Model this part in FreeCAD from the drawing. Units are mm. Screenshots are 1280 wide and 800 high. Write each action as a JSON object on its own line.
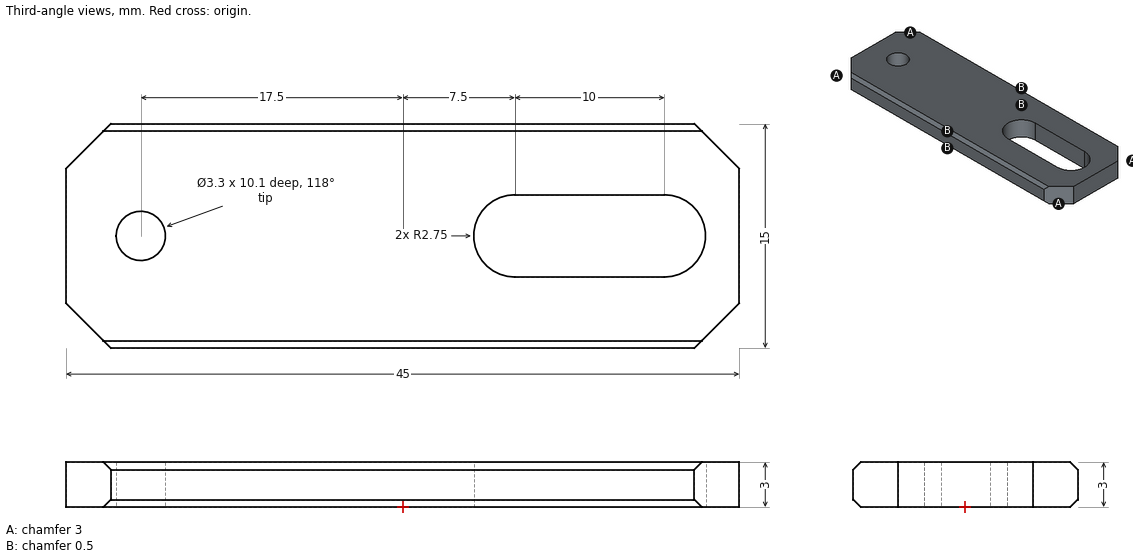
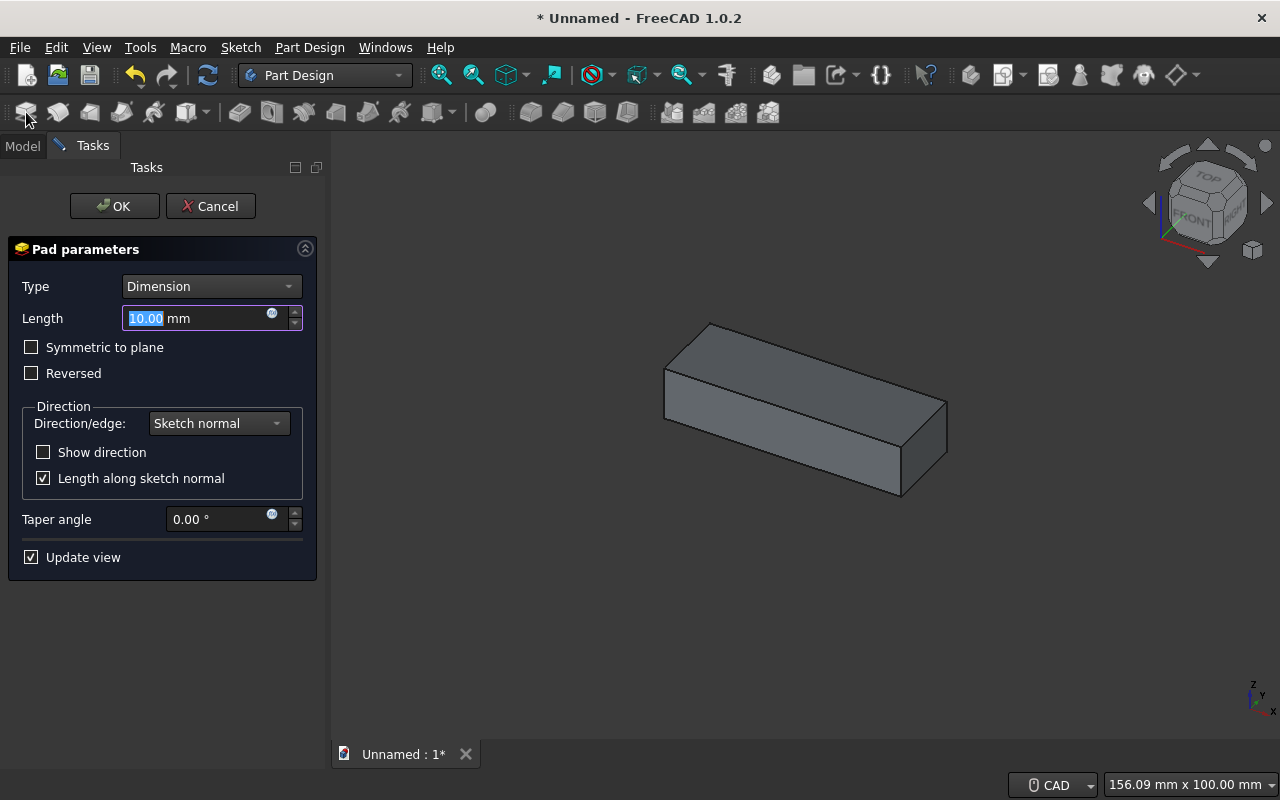
{"action": "type", "text": "3"}
{"action": "key", "text": "Tab"}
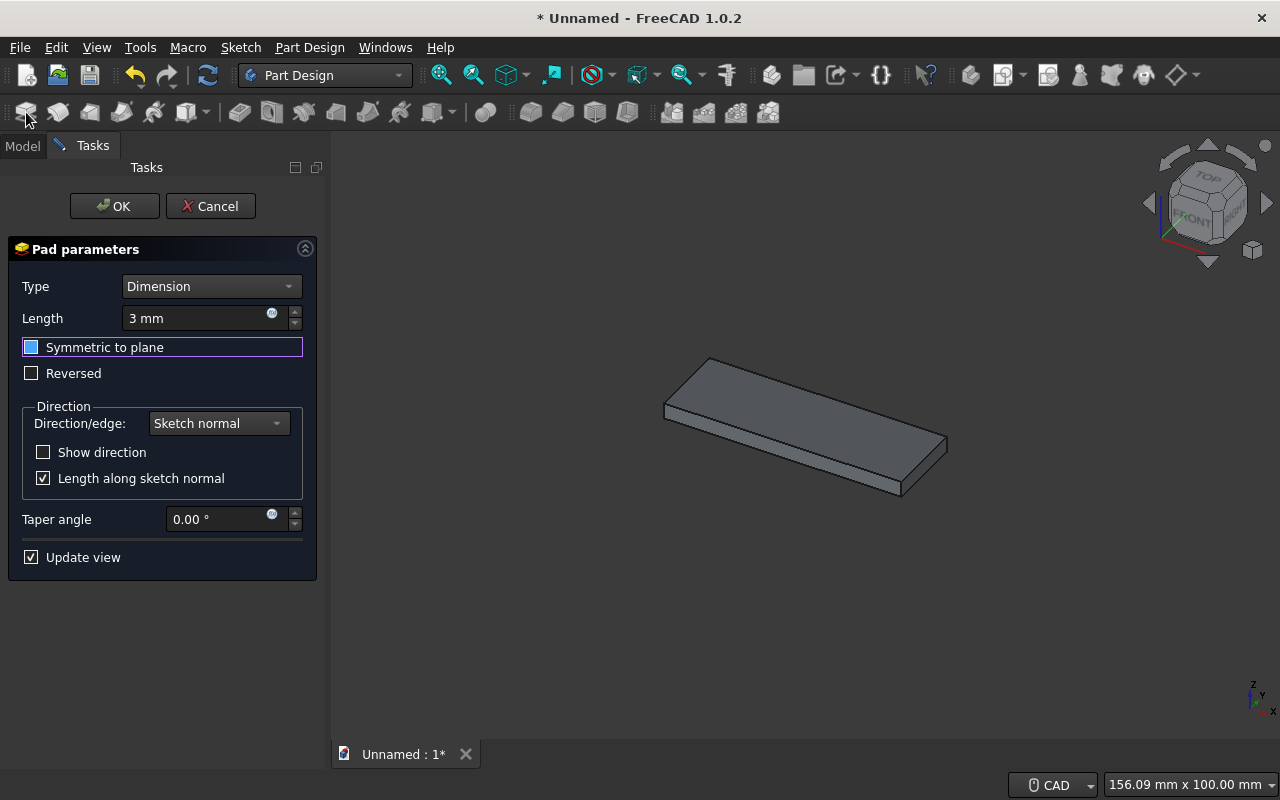
{"action": "left_click", "coordinate": [115, 206]}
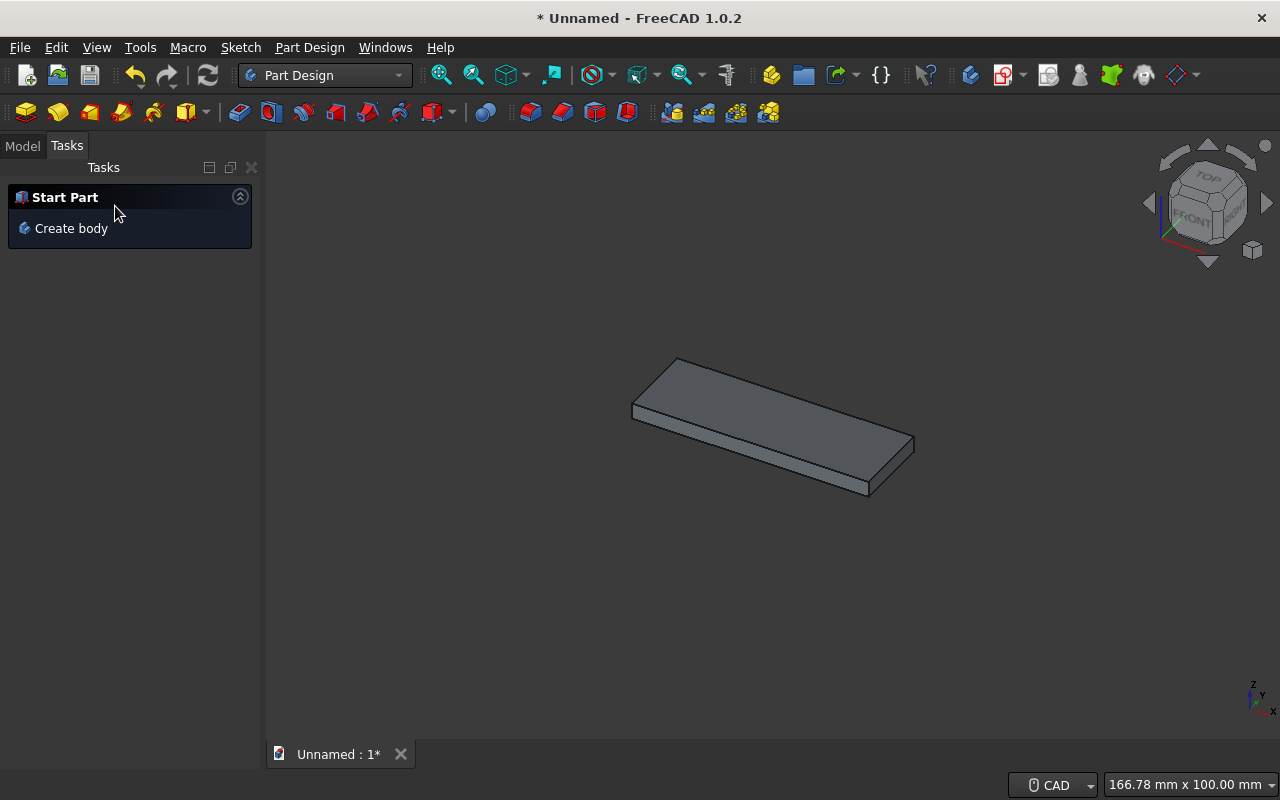
{"action": "left_click", "coordinate": [442, 76]}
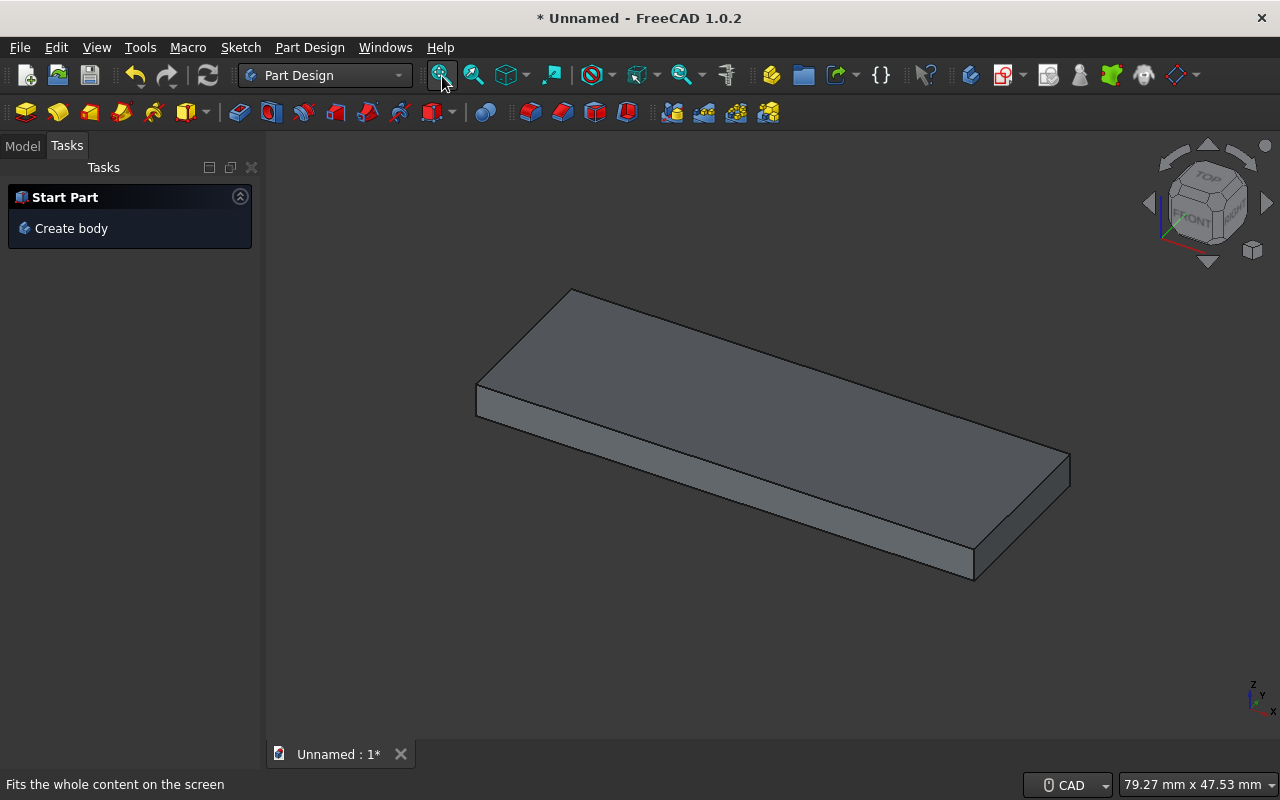
{"action": "left_click", "coordinate": [915, 465]}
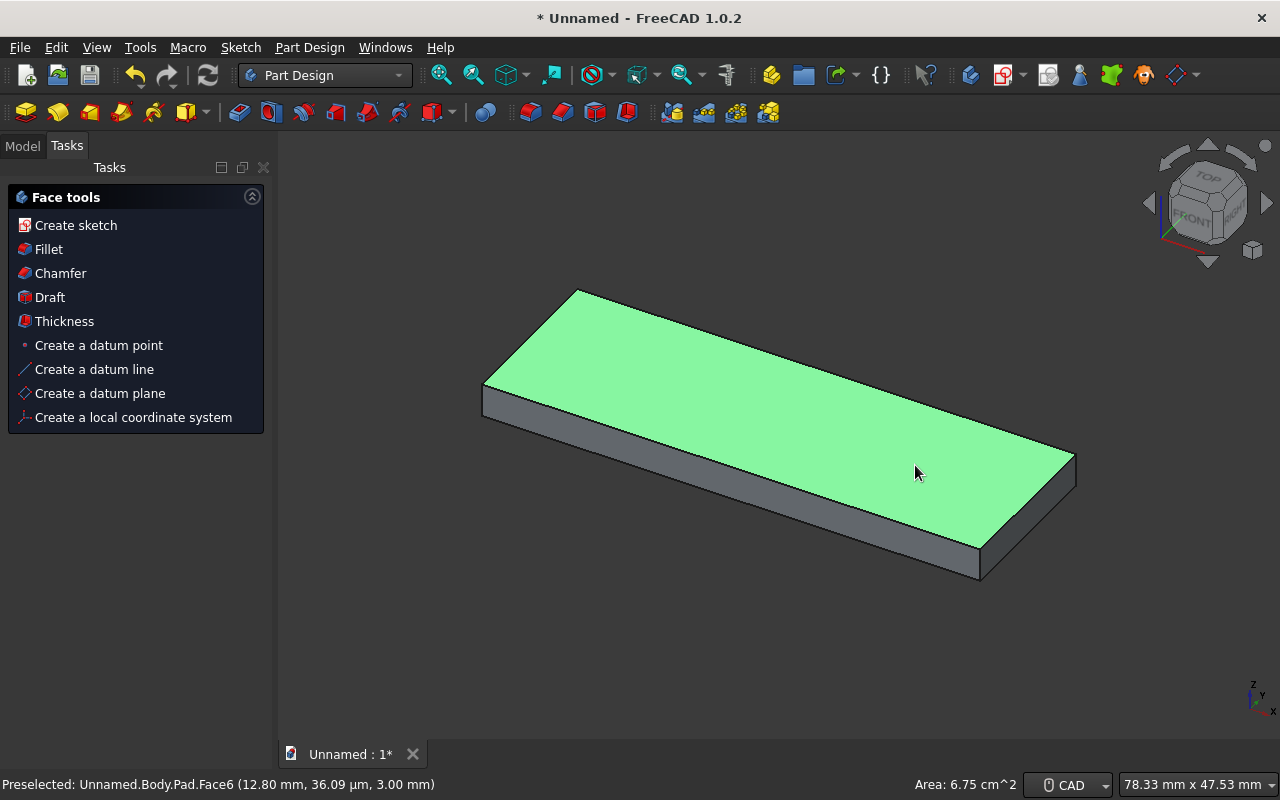
{"action": "left_click", "coordinate": [1004, 76]}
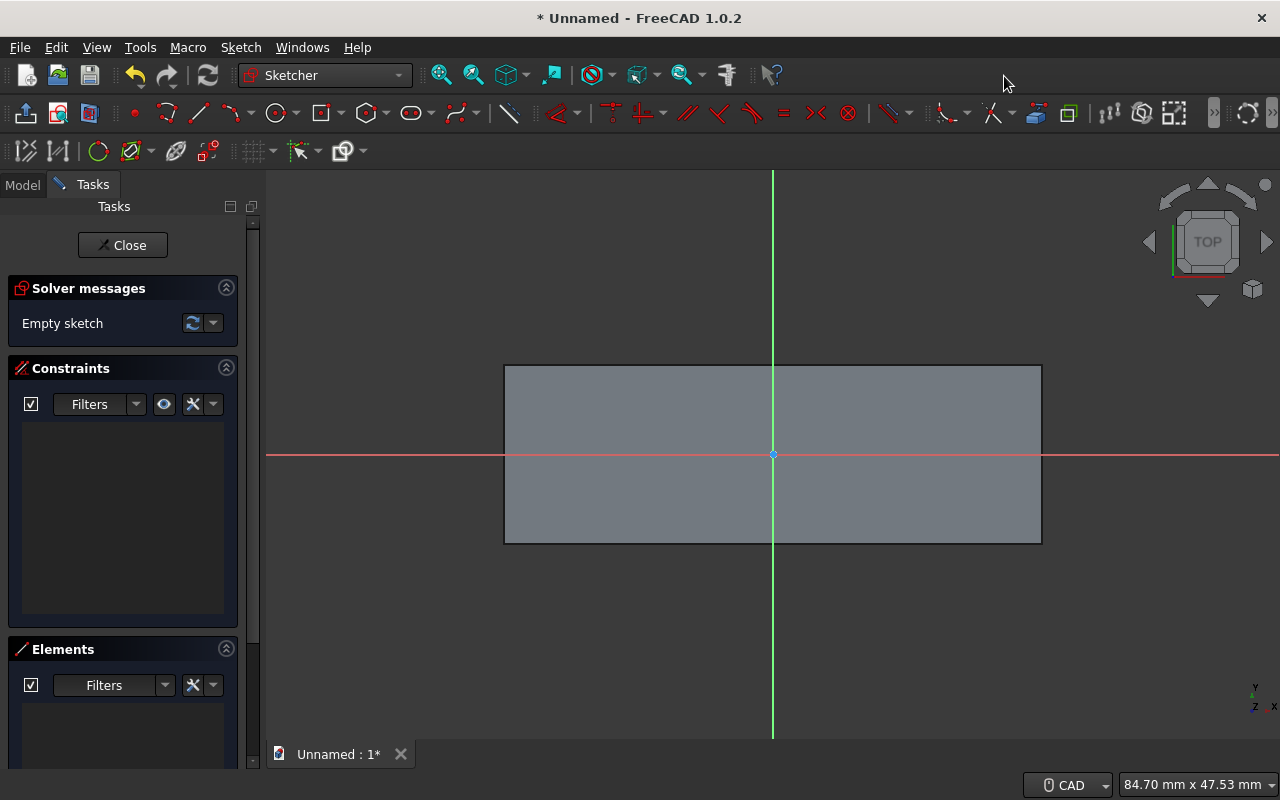
{"action": "scroll", "coordinate": [546, 454], "scroll_direction": "up", "scroll_amount": 11}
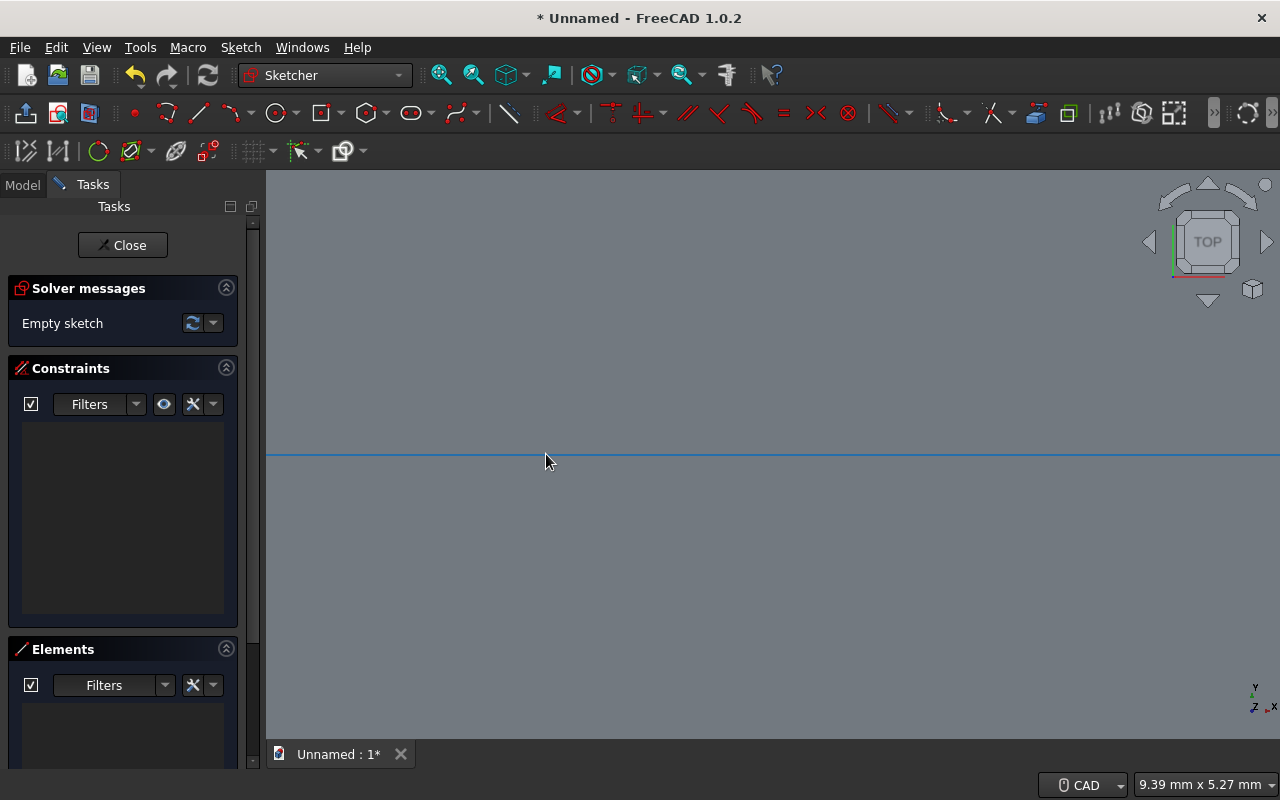
{"action": "left_click", "coordinate": [276, 114]}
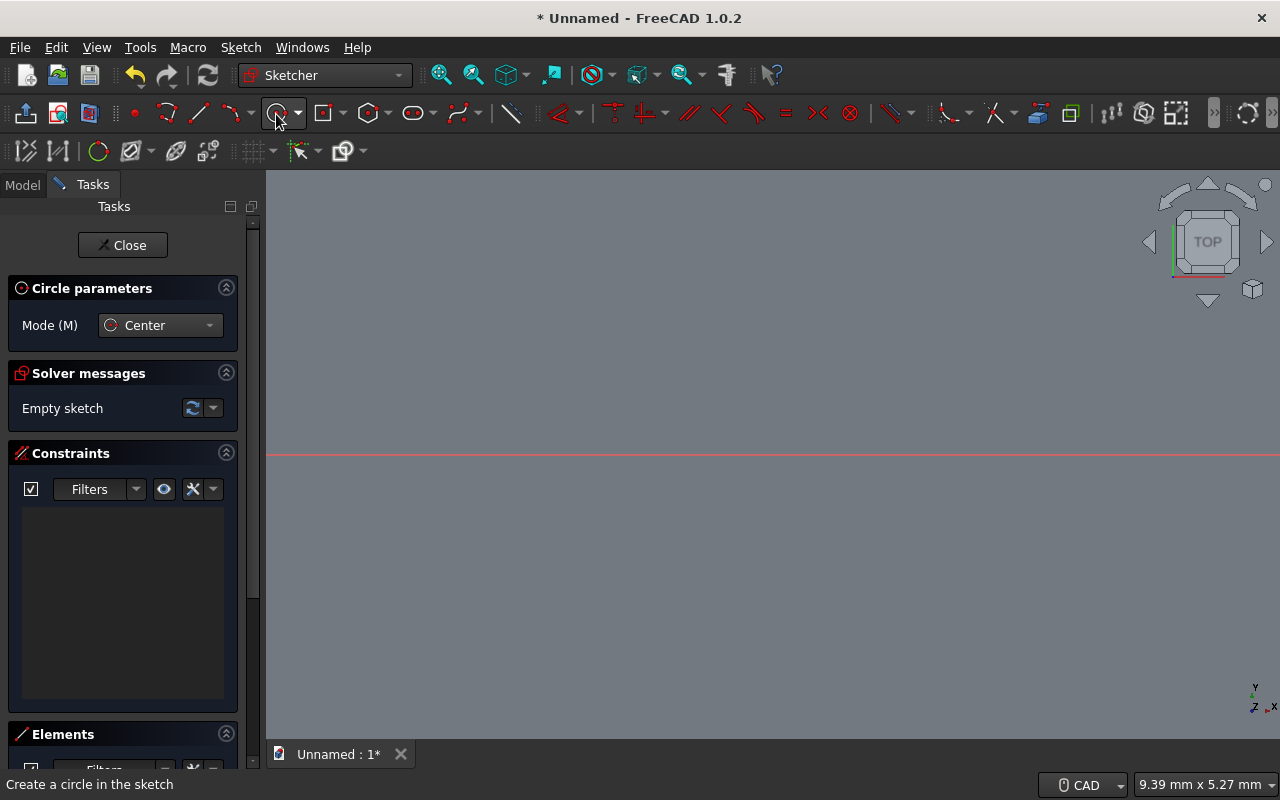
{"action": "left_click", "coordinate": [702, 454]}
{"action": "mouse_move", "coordinate": [828, 328]}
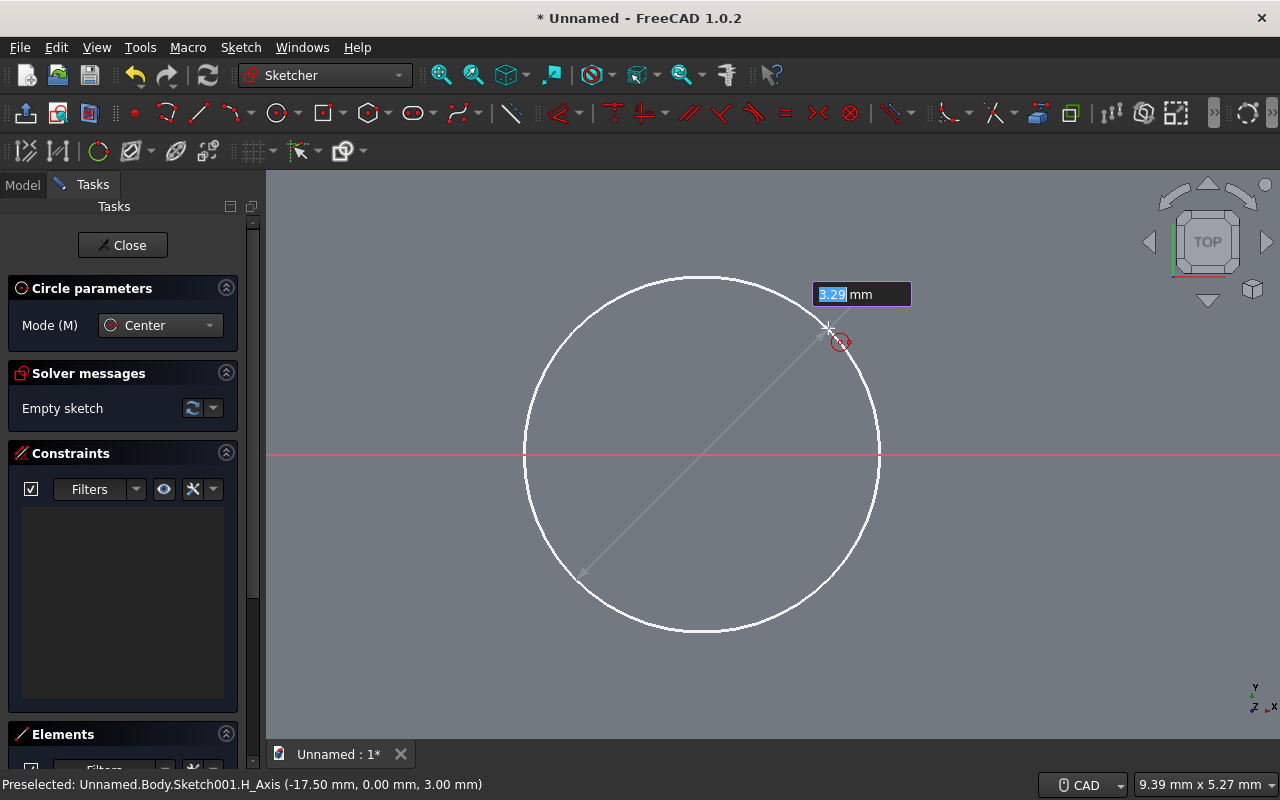
{"action": "type", "text": "3.3"}
{"action": "key", "text": "Return"}
{"action": "key", "text": "Escape"}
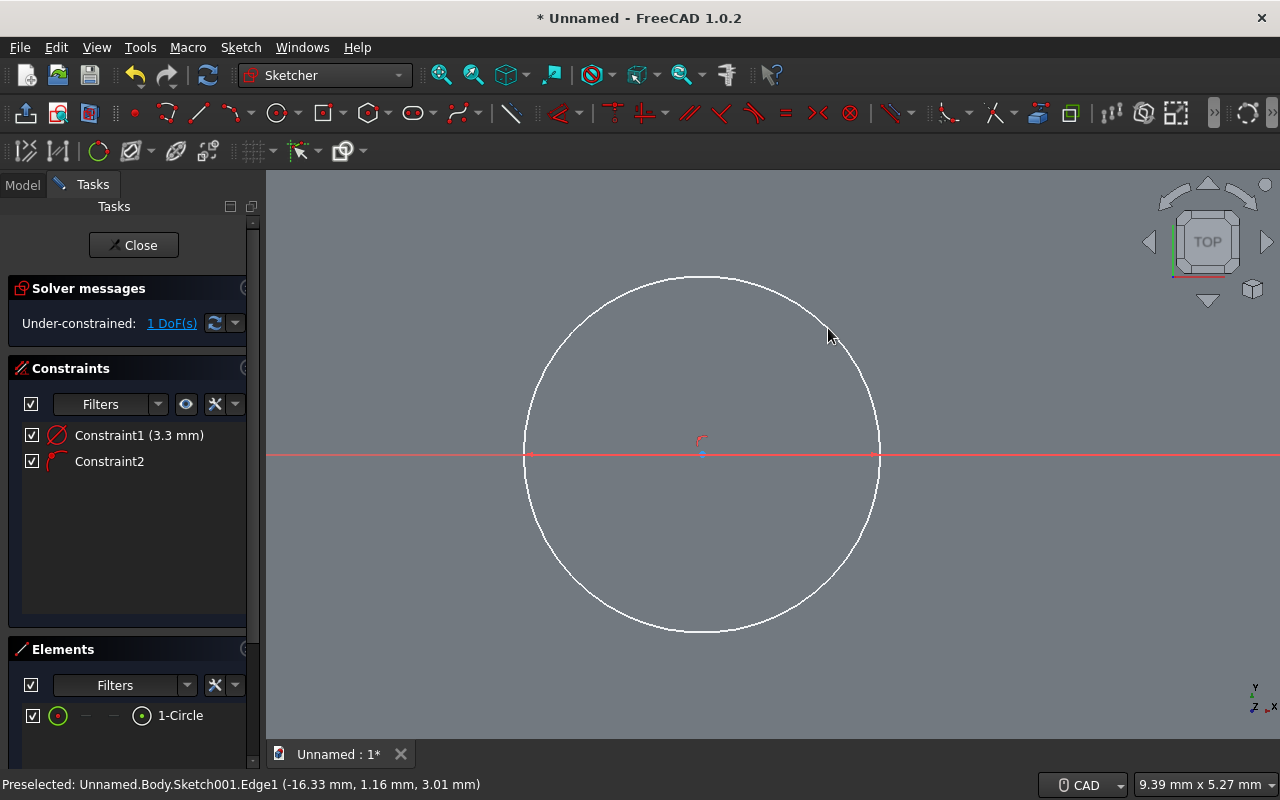
{"action": "left_click", "coordinate": [702, 454]}